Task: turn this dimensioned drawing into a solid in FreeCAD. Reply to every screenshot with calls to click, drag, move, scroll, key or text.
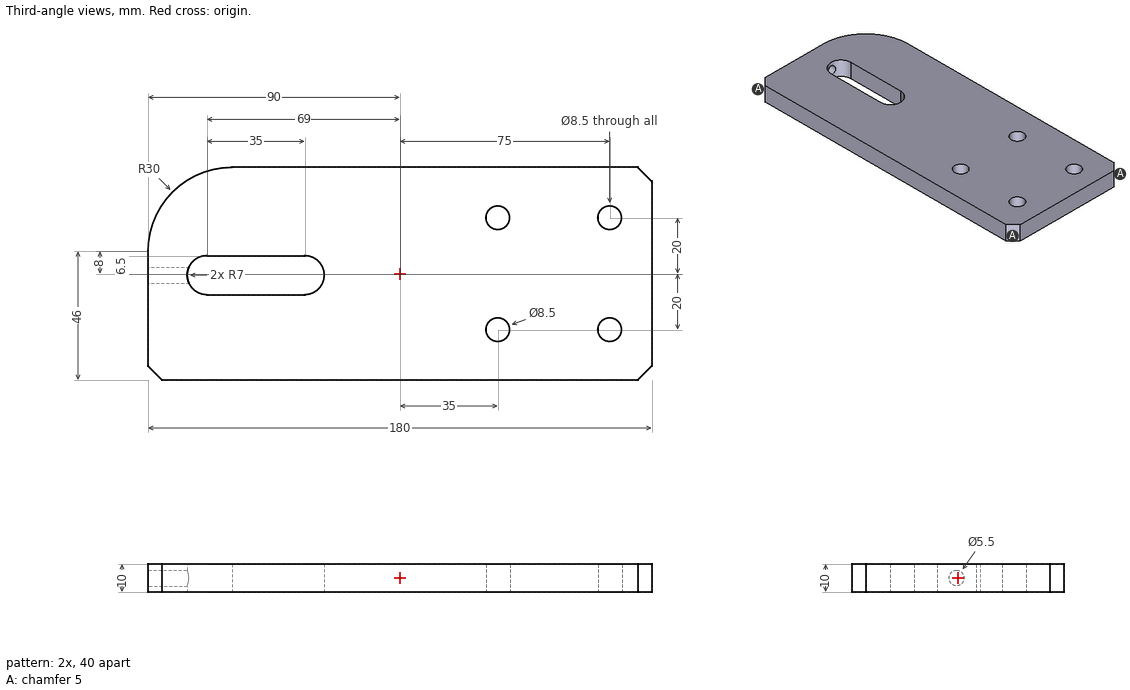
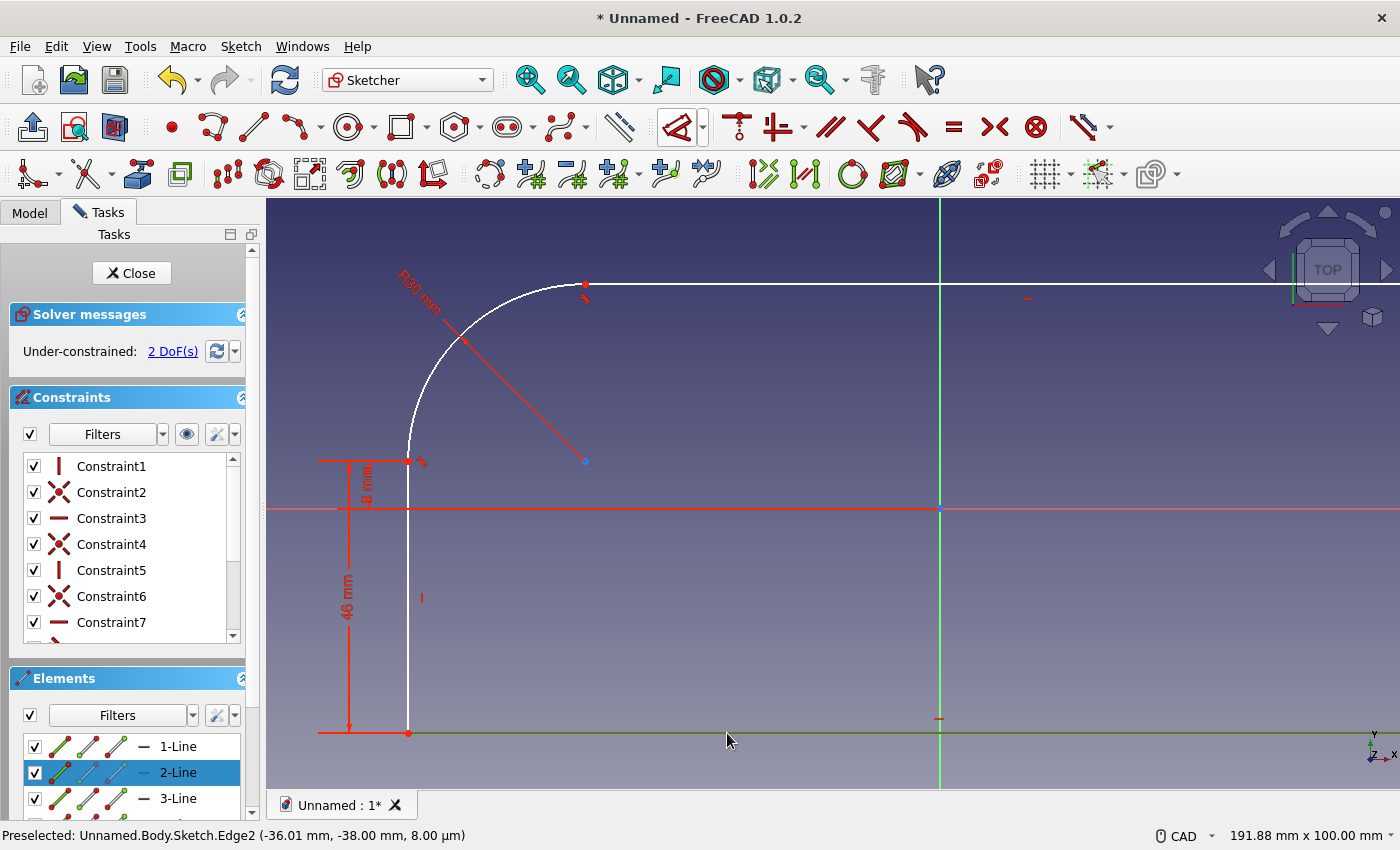
key(l)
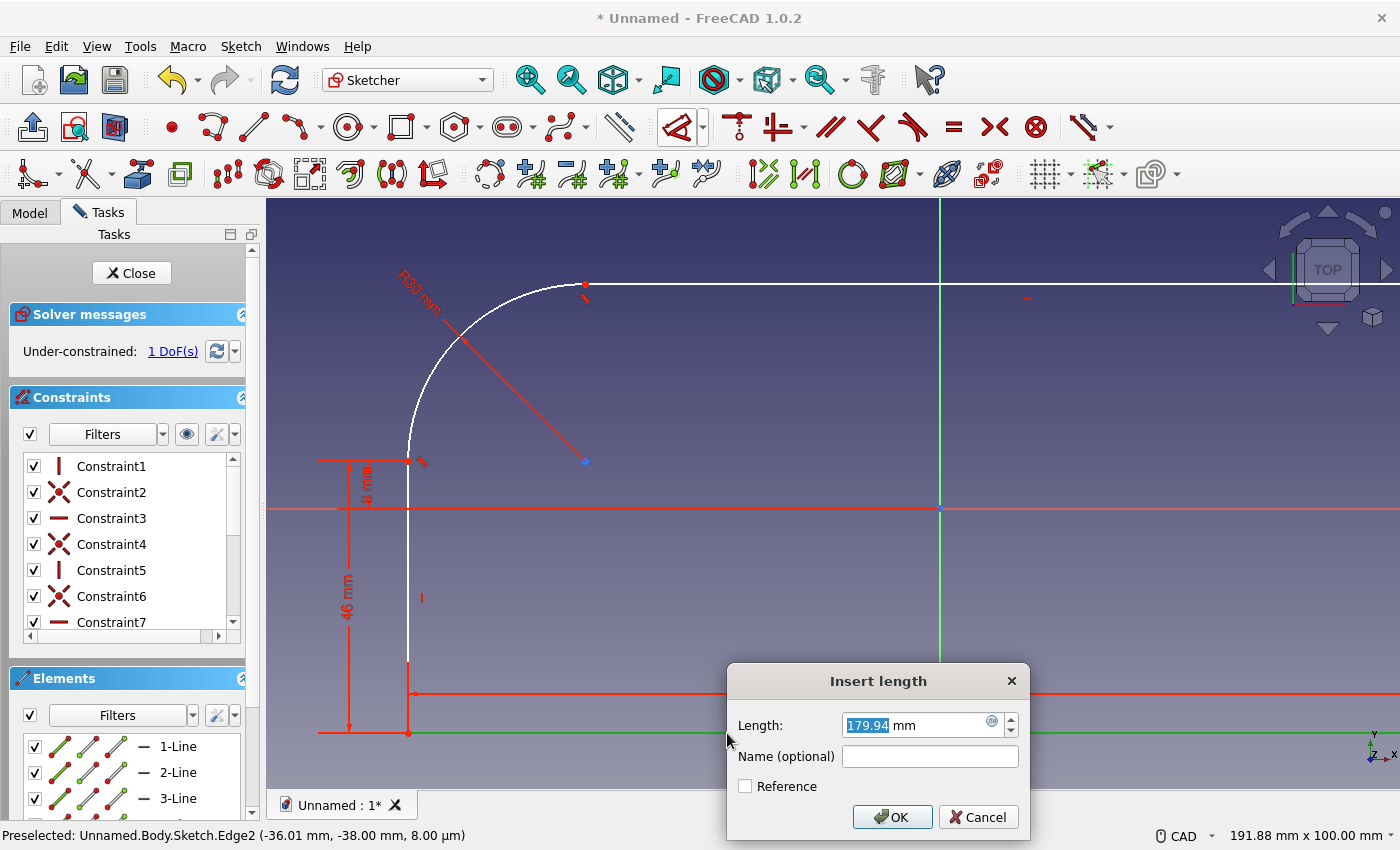
text(180)
key(Return)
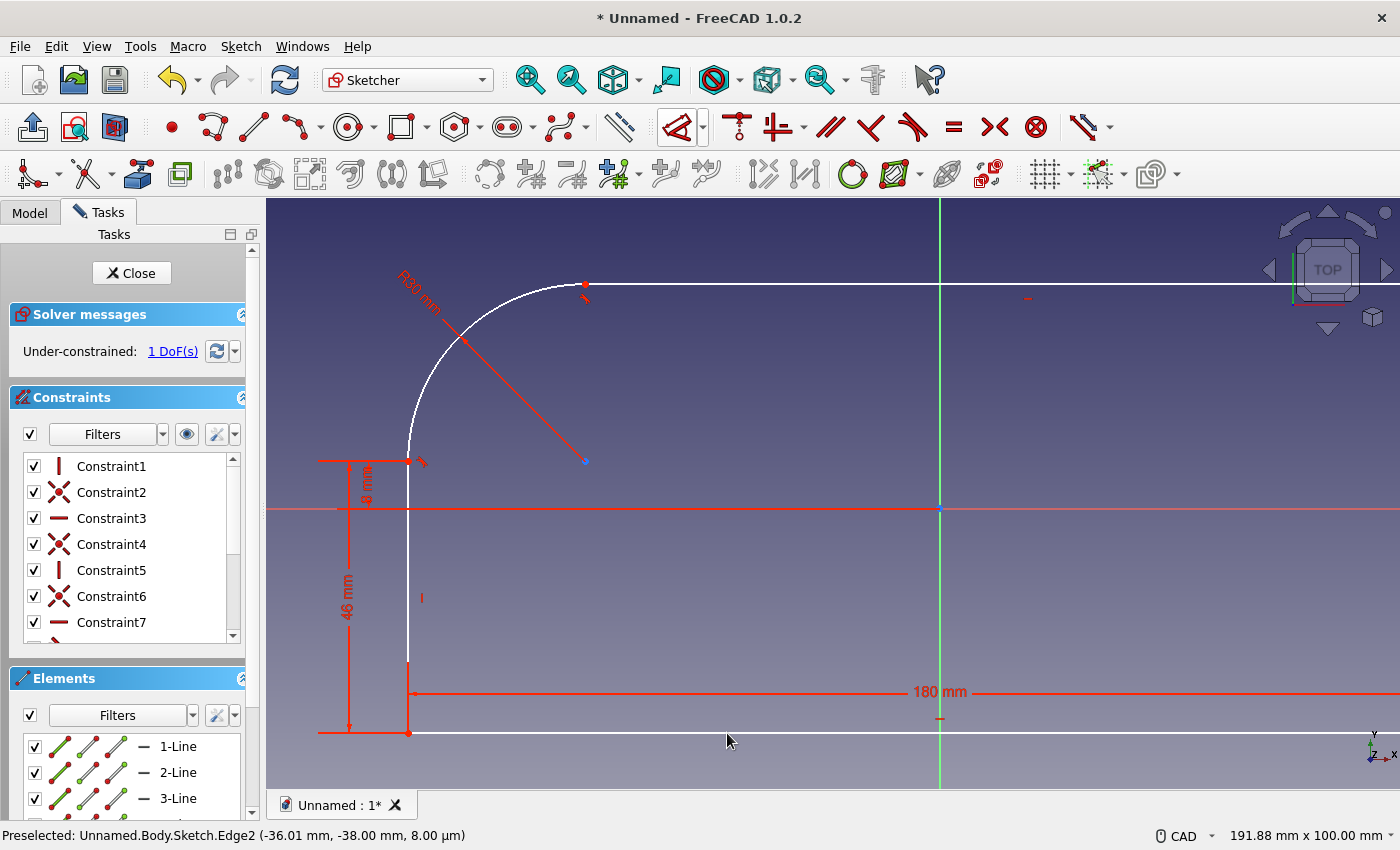
click(408, 461)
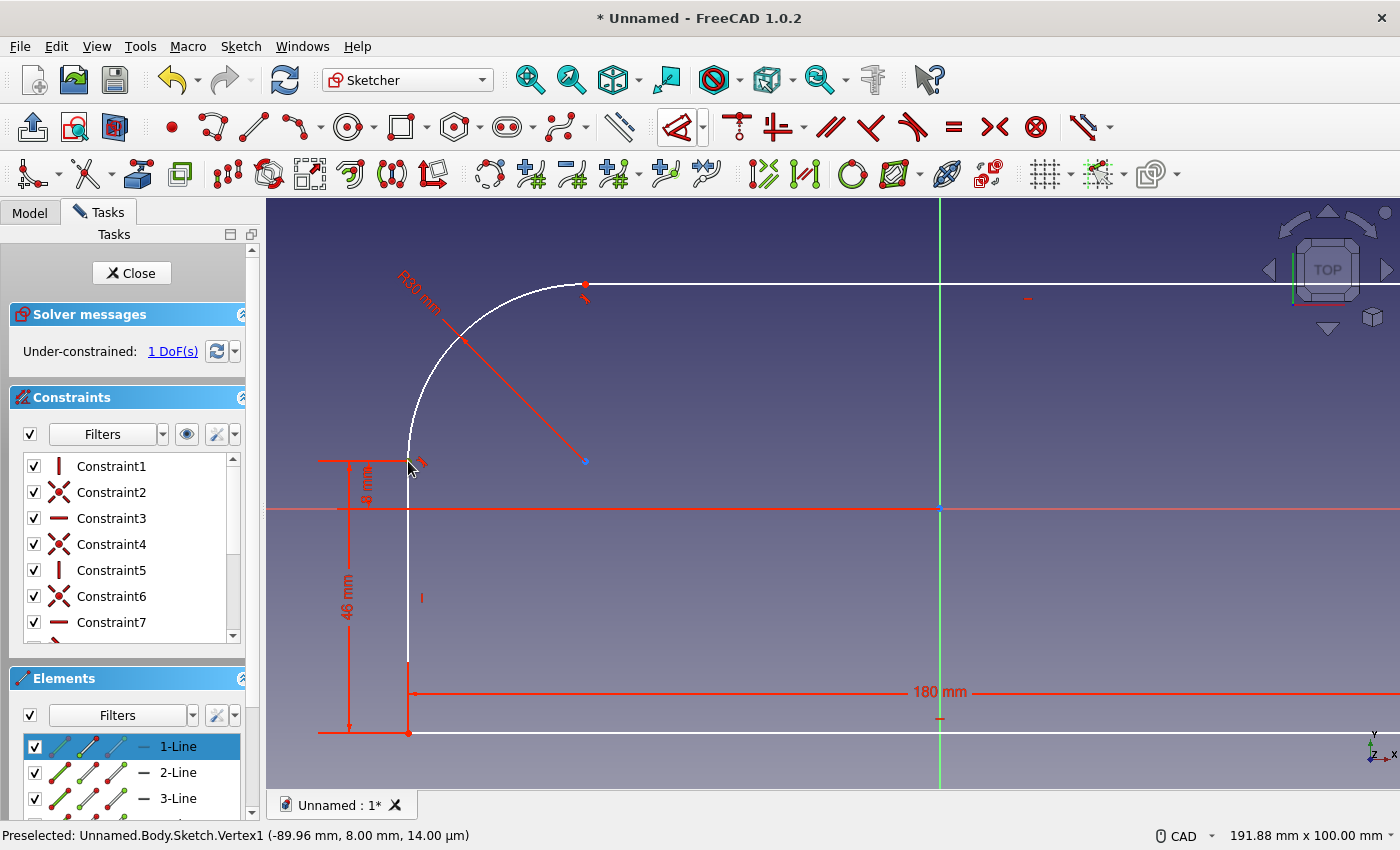
click(702, 128)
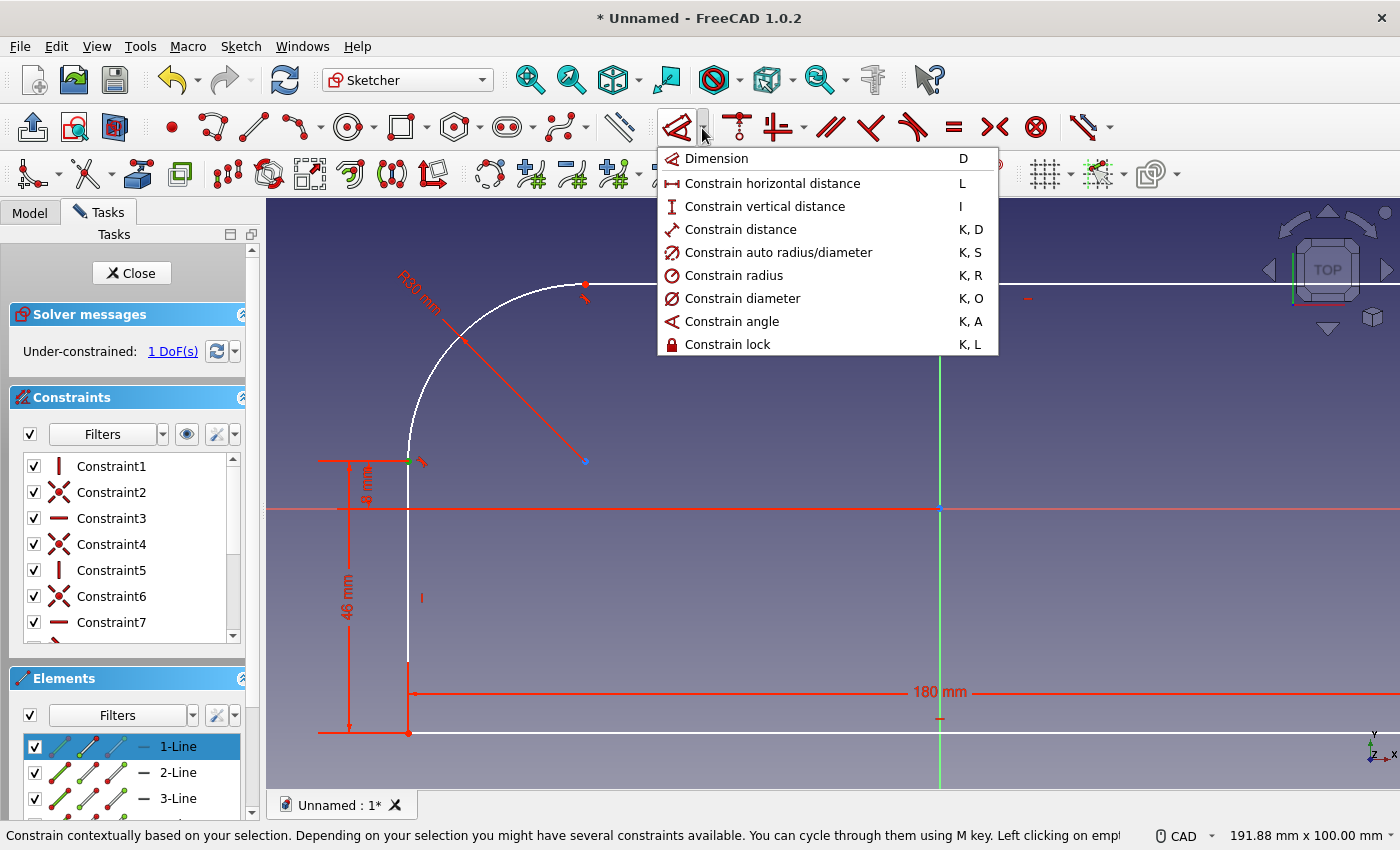
click(828, 184)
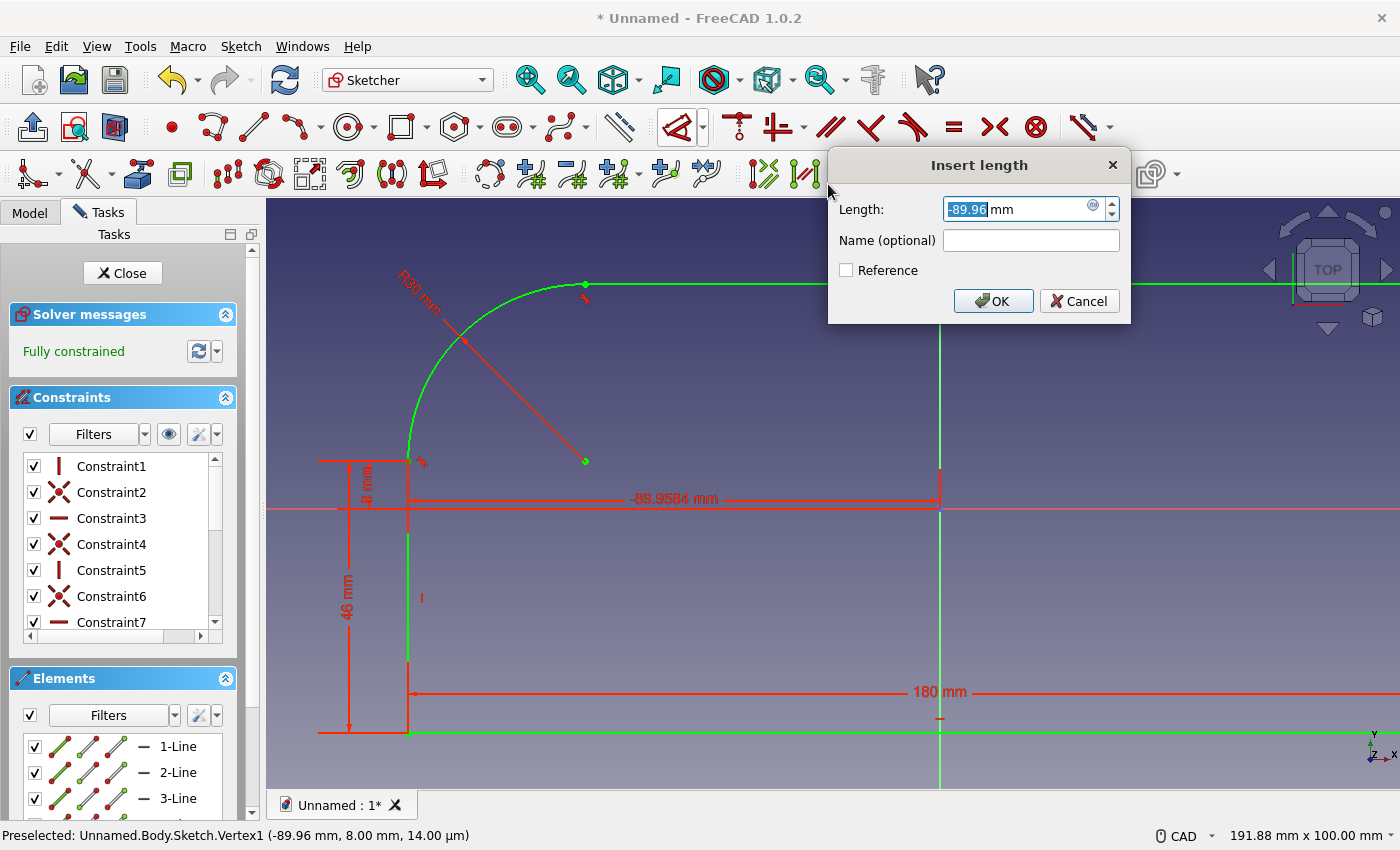
text(-90)
key(Return)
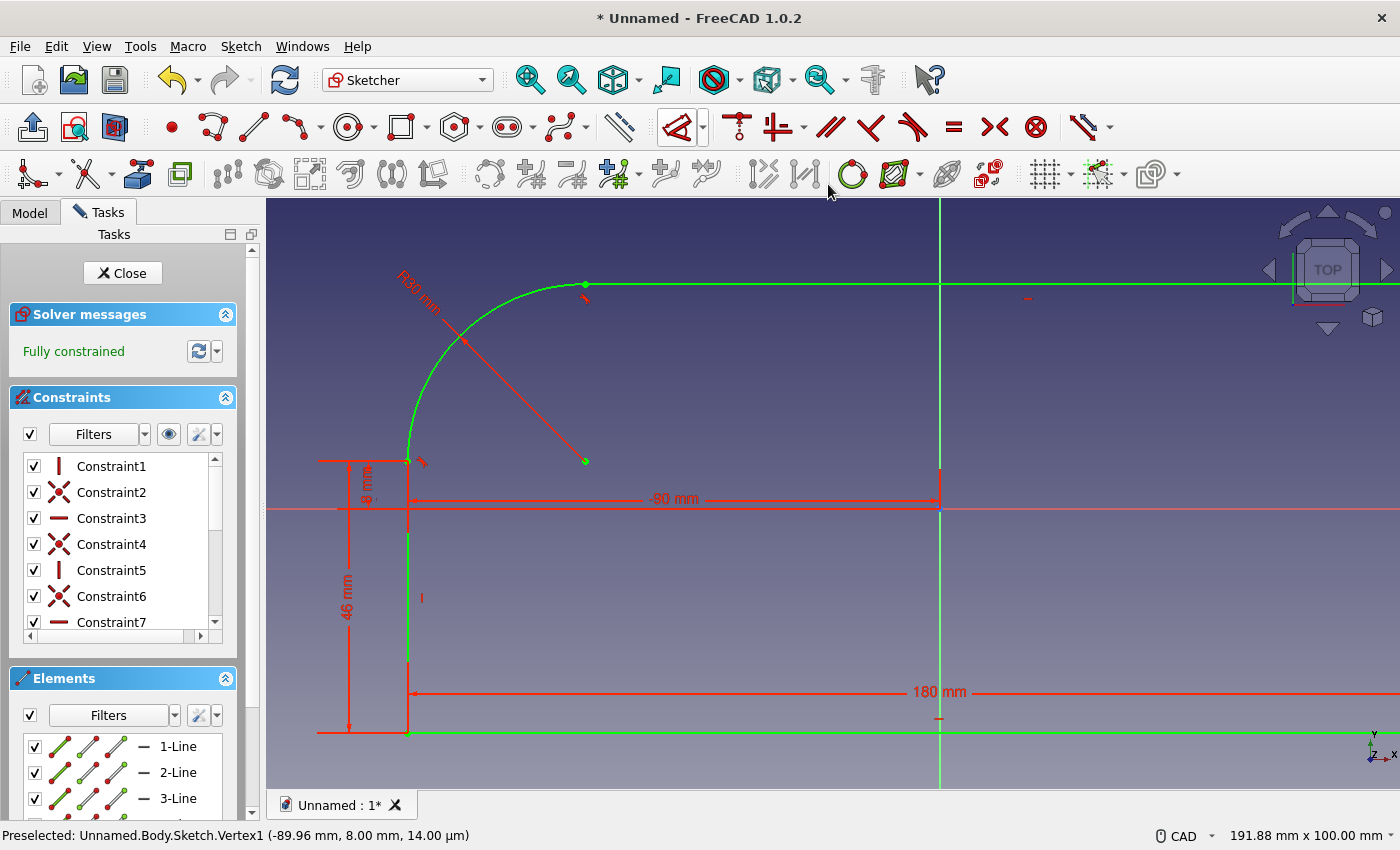
click(123, 273)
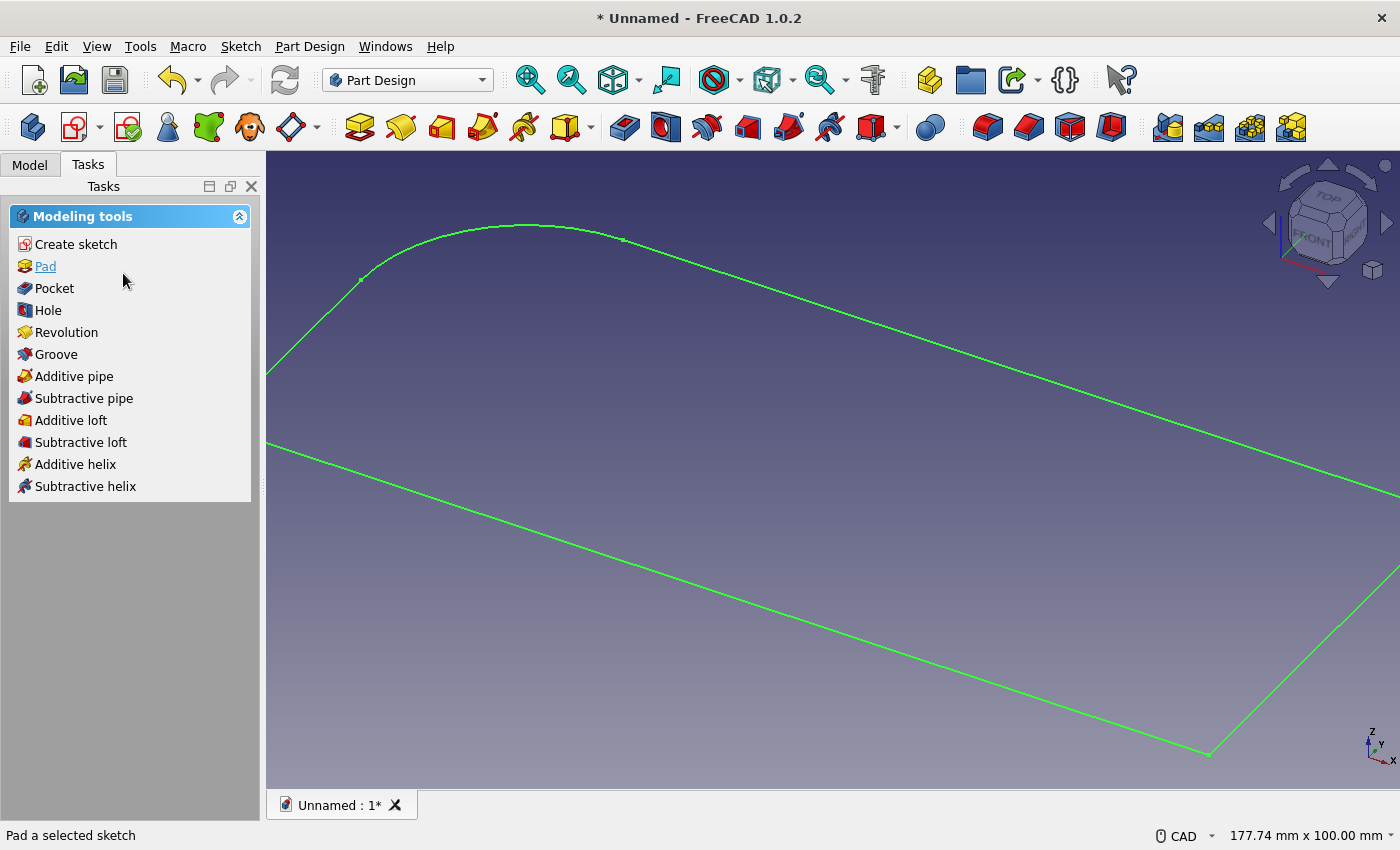
click(360, 128)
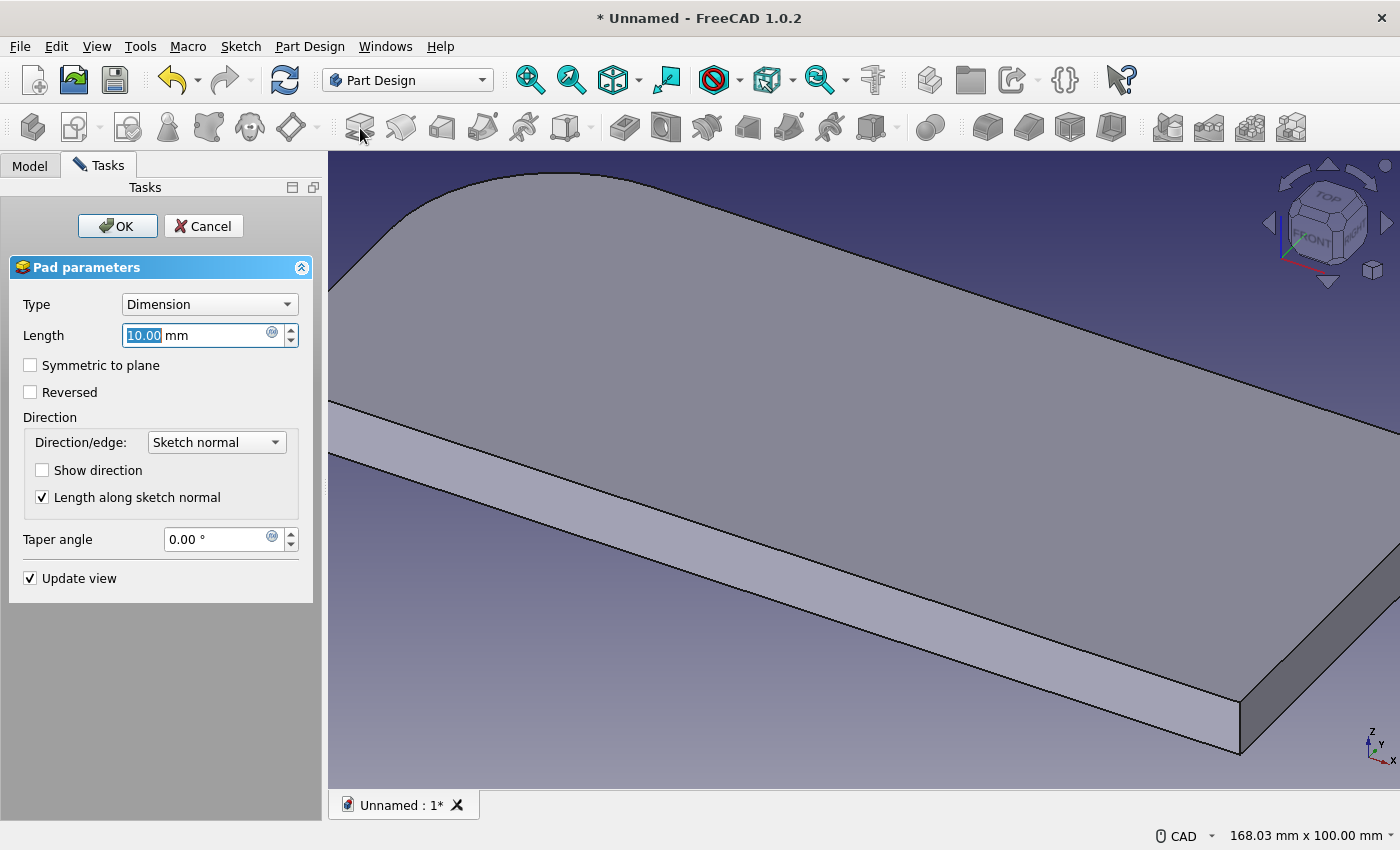
text(10)
key(Tab)